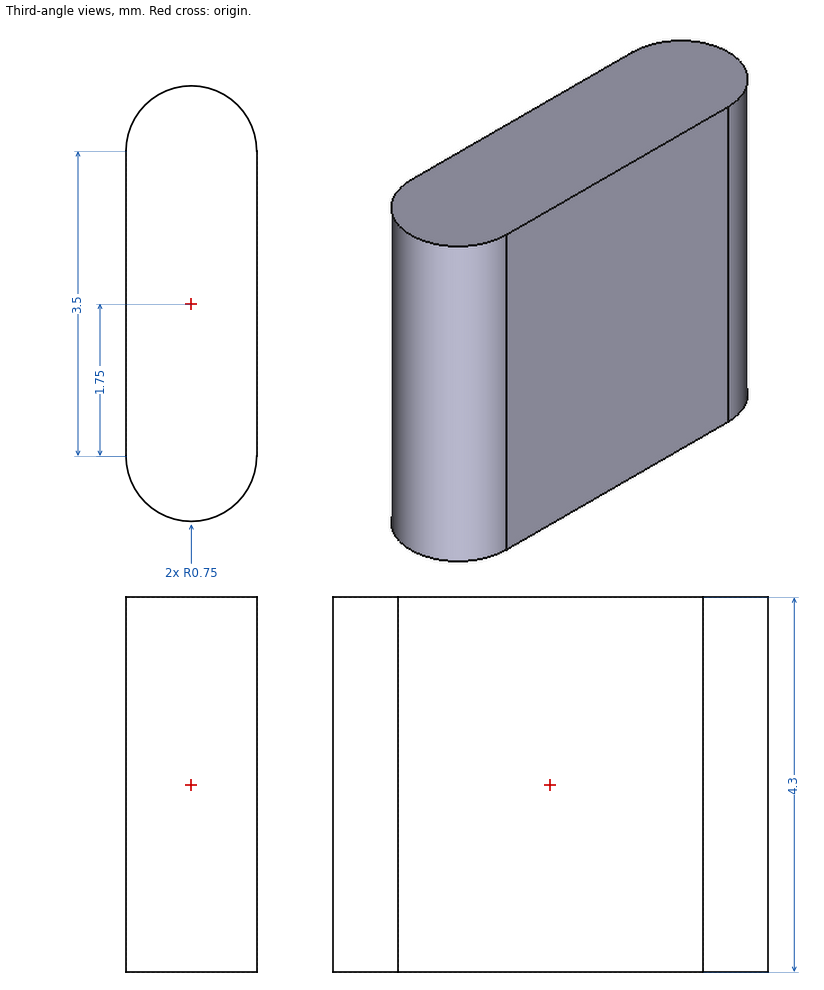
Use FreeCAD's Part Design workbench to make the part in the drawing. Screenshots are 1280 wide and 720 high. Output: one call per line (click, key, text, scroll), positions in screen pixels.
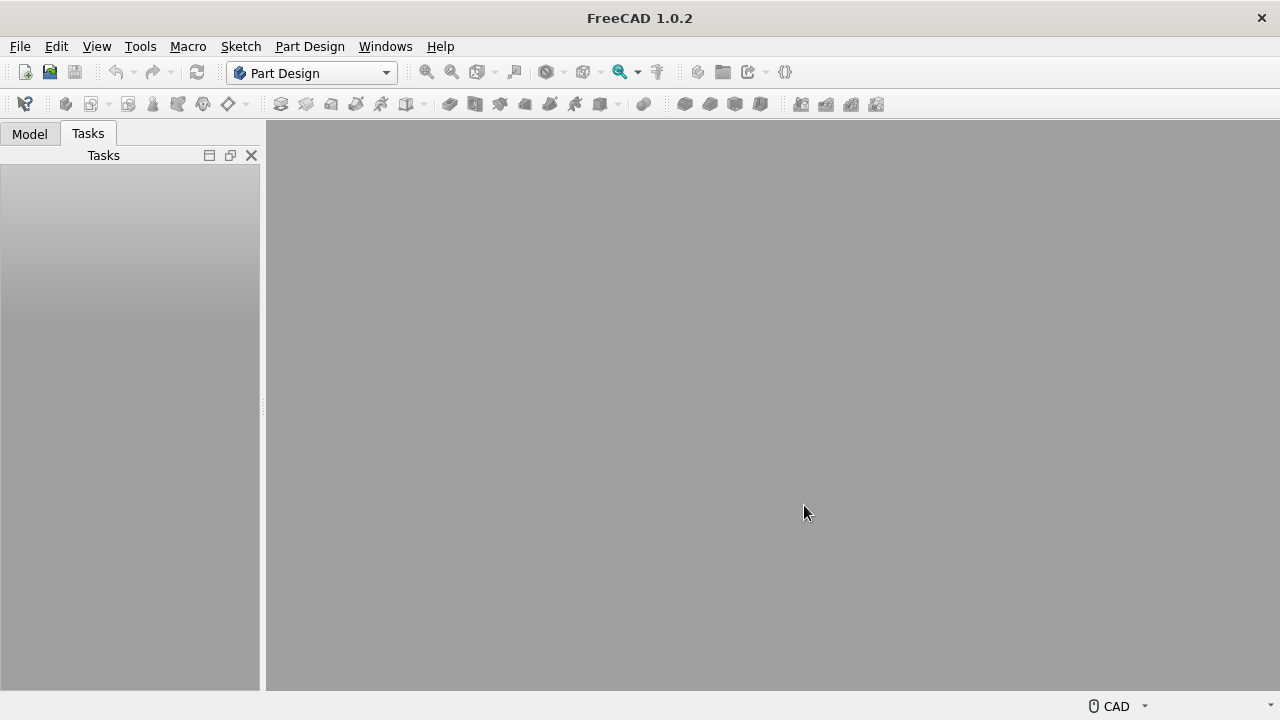
click(25, 72)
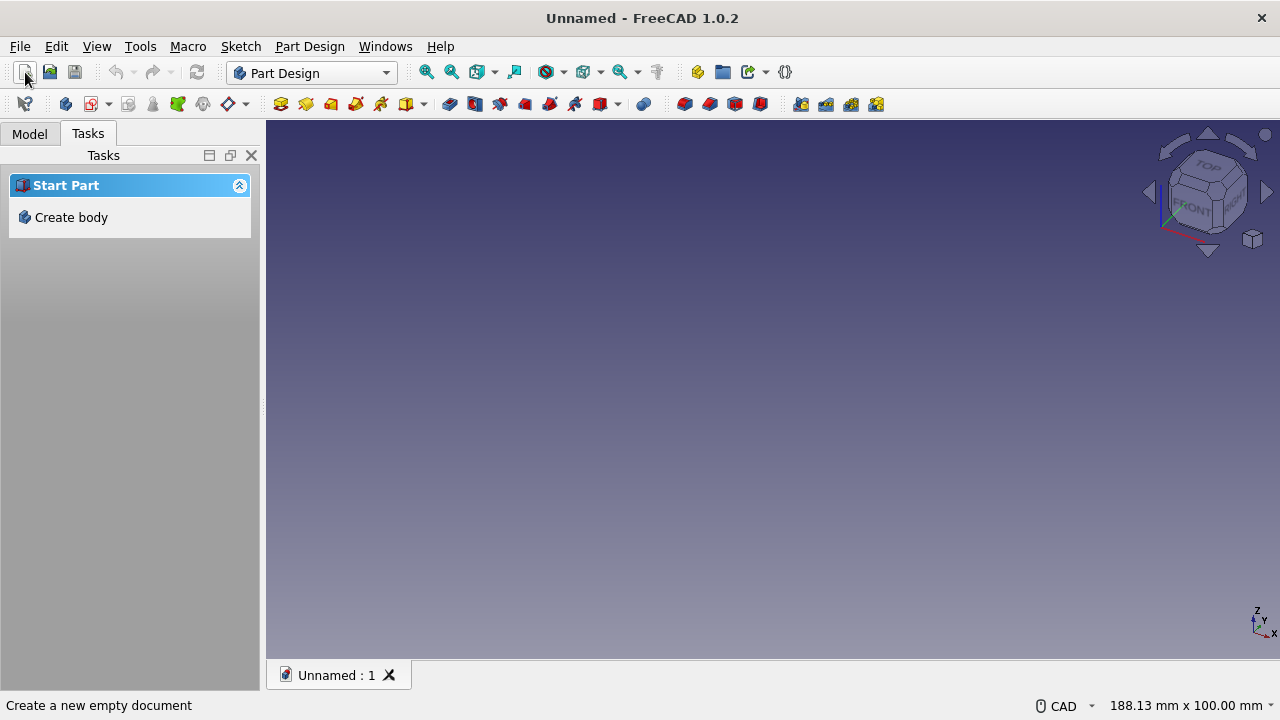
click(90, 104)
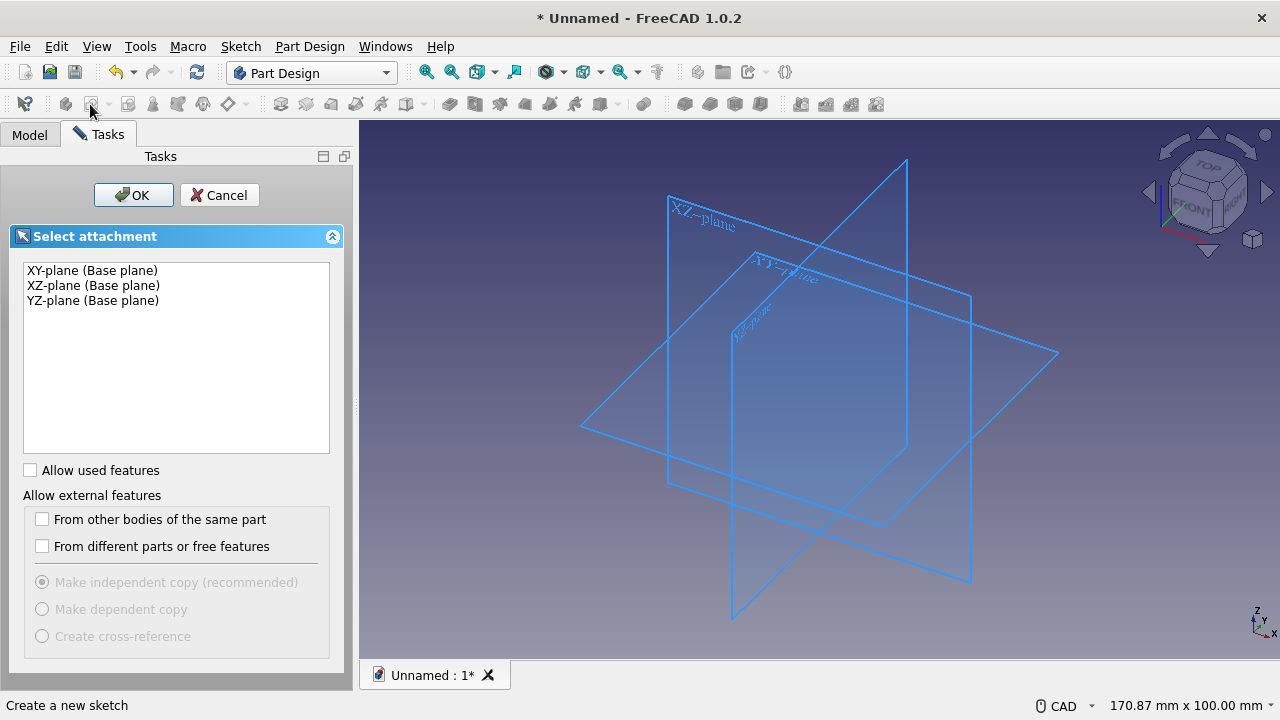
click(84, 270)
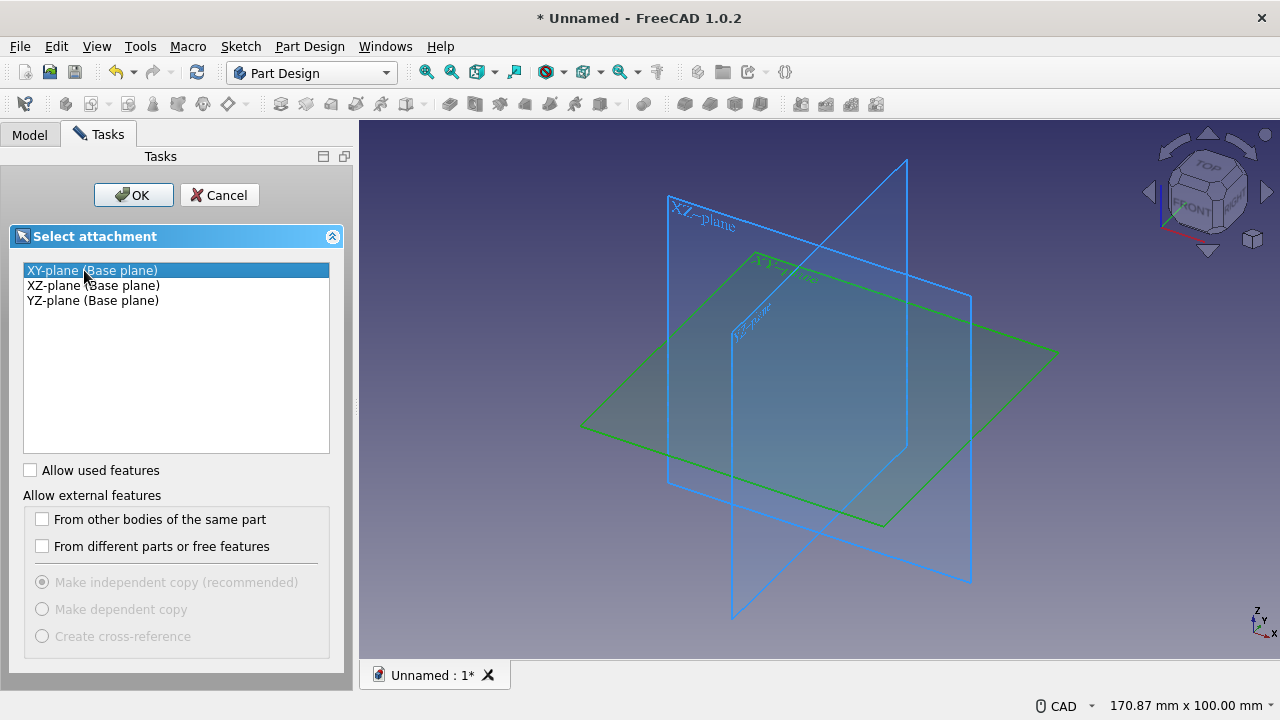
click(134, 195)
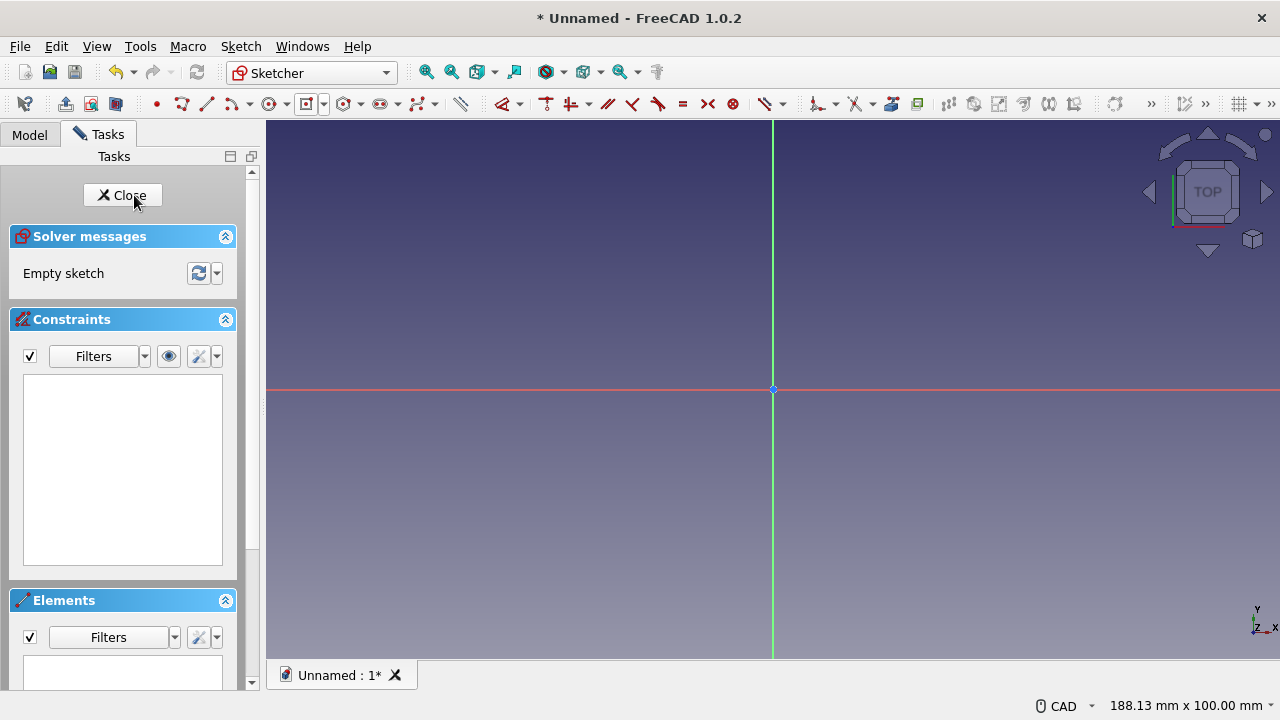
scroll(778, 390, up, 13)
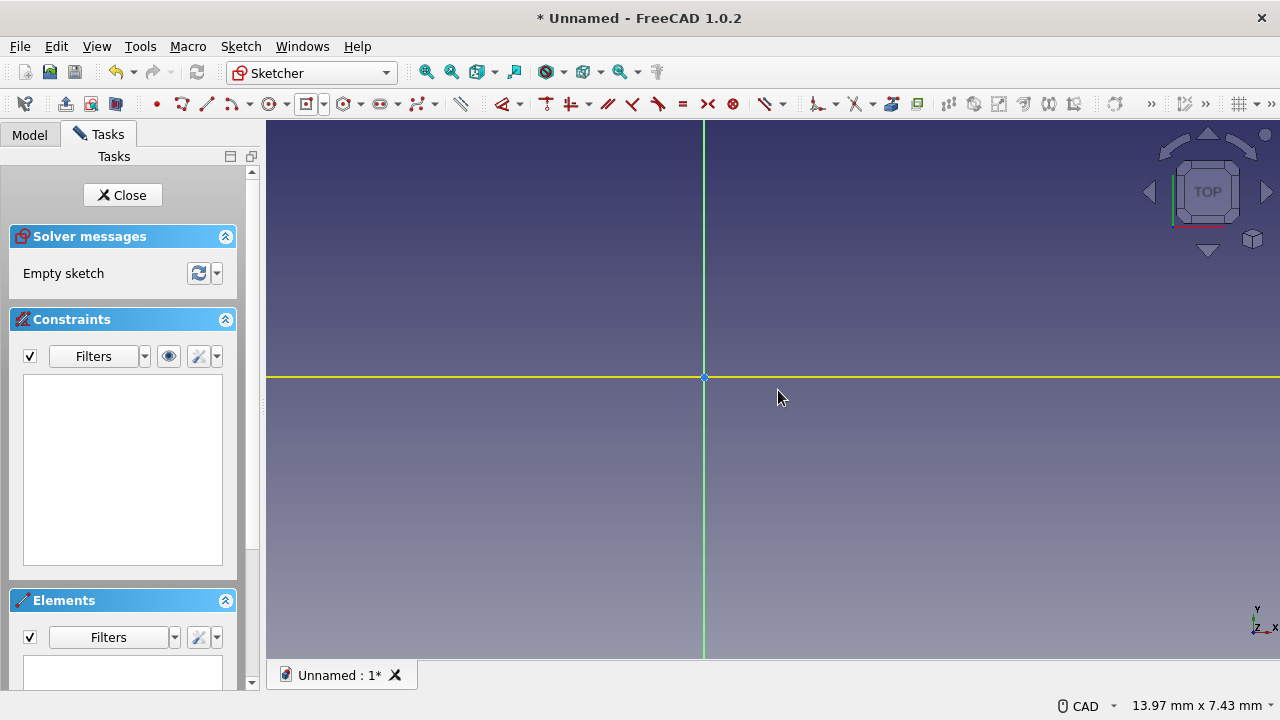
click(380, 104)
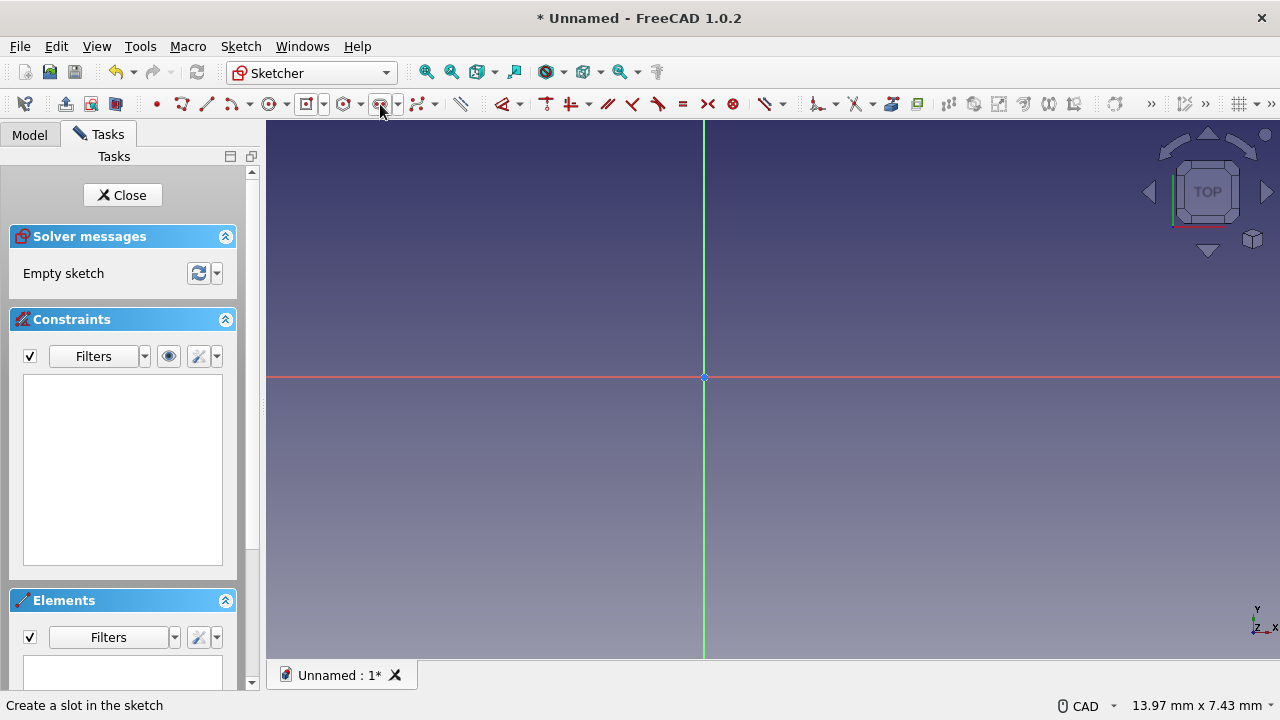
click(704, 504)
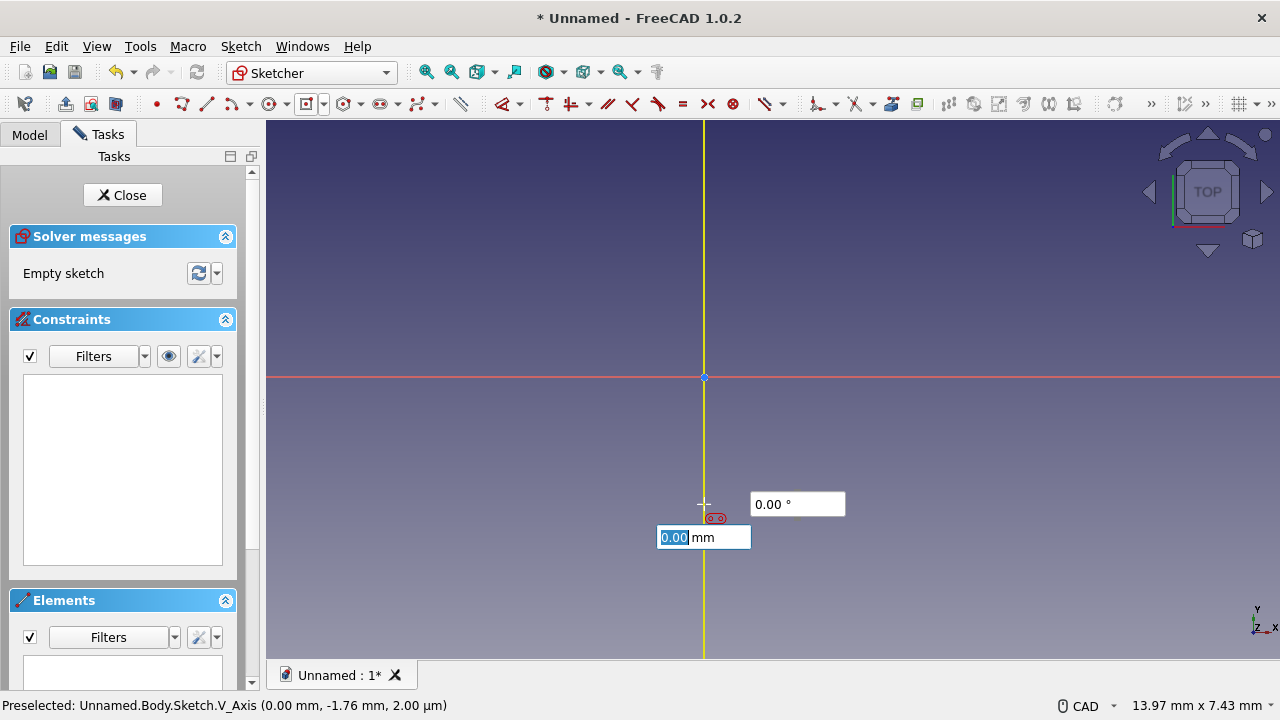
click(713, 250)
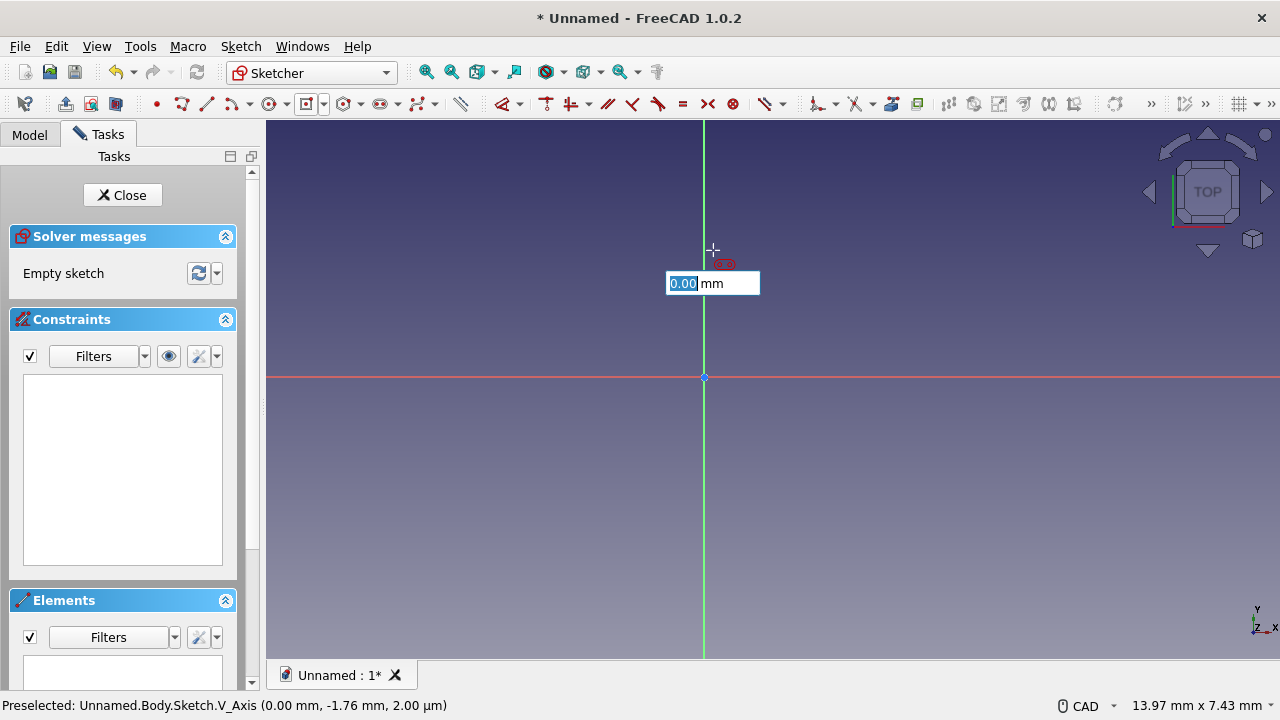
click(650, 339)
key(Escape)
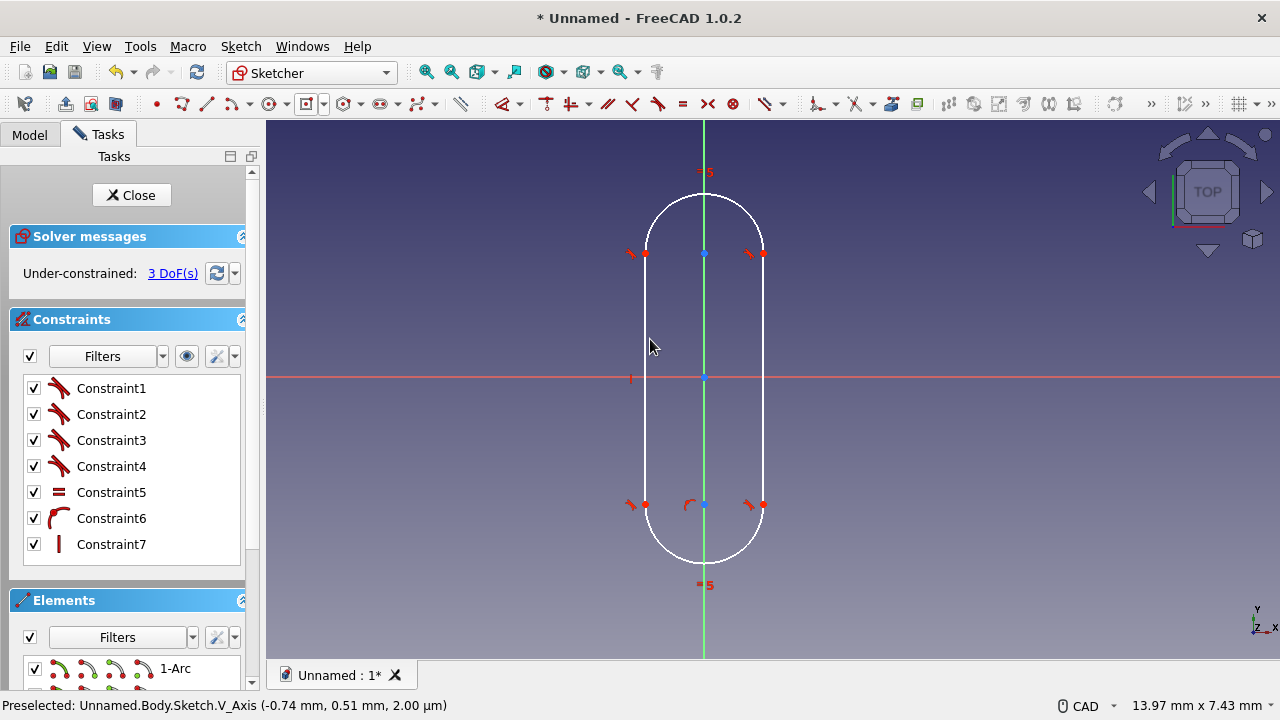
click(502, 104)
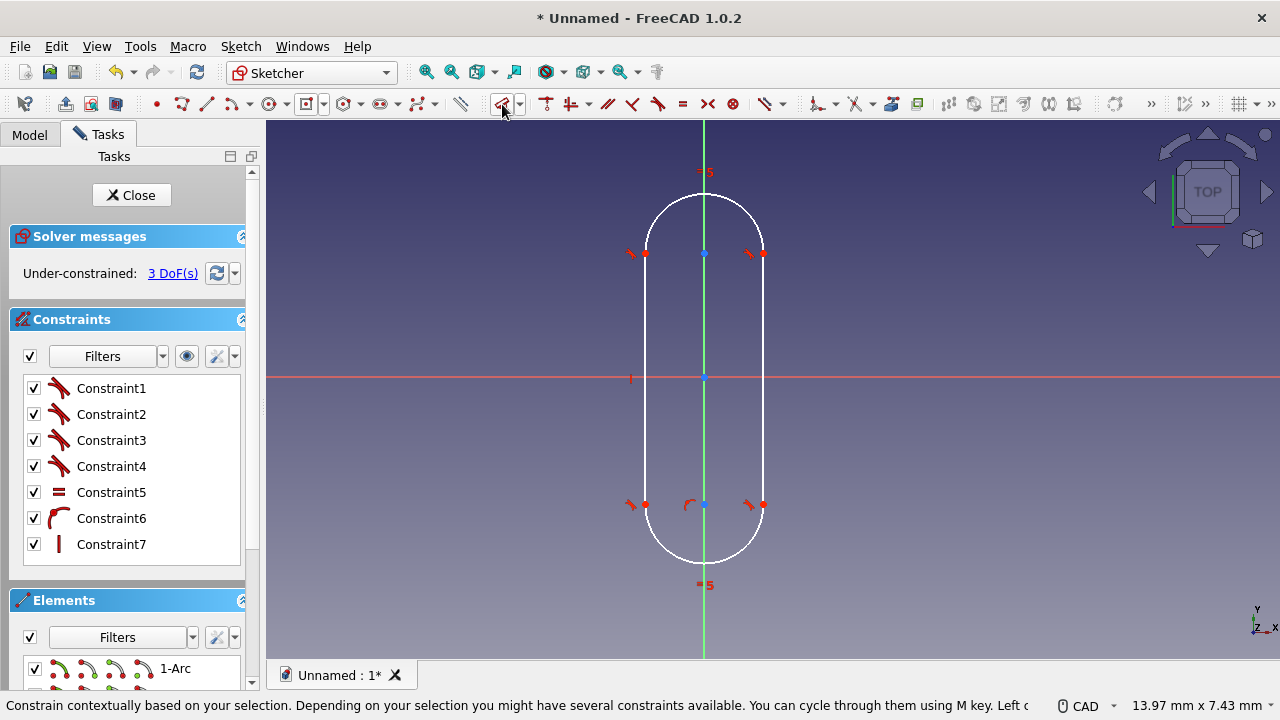
click(670, 552)
click(651, 578)